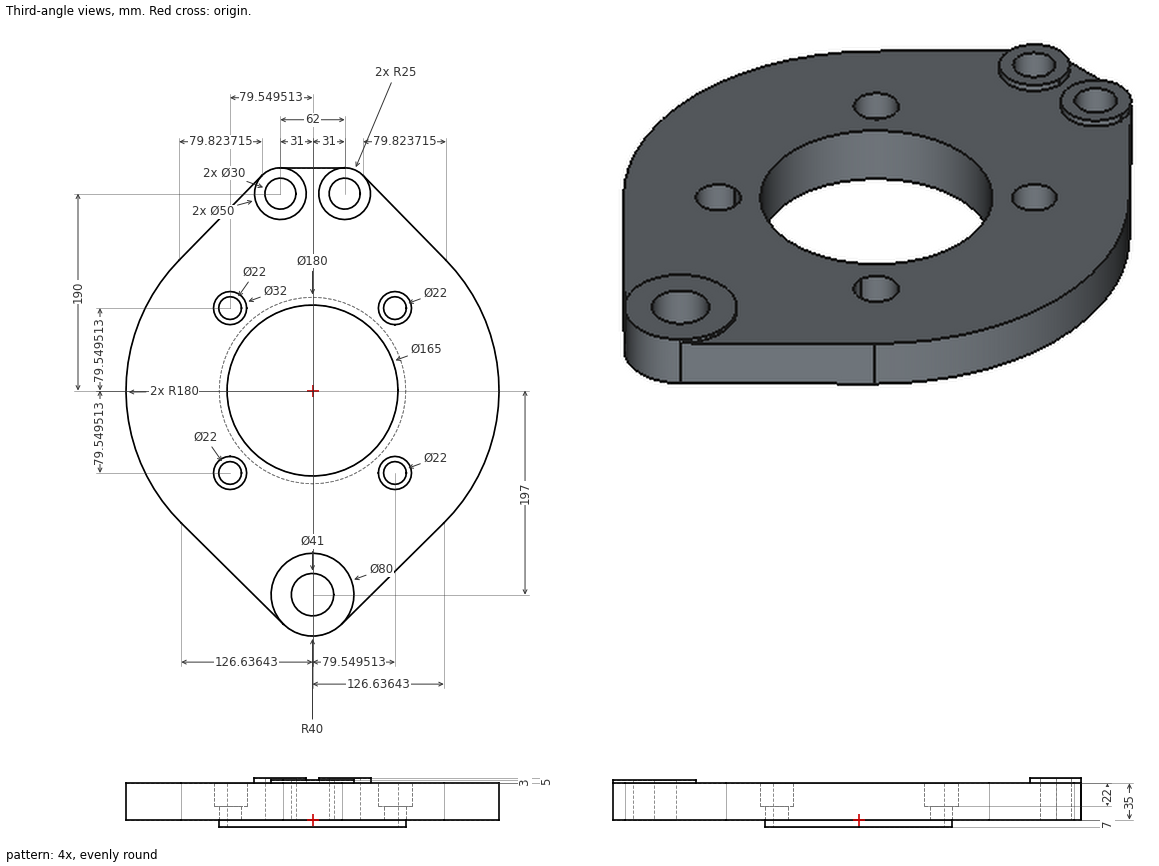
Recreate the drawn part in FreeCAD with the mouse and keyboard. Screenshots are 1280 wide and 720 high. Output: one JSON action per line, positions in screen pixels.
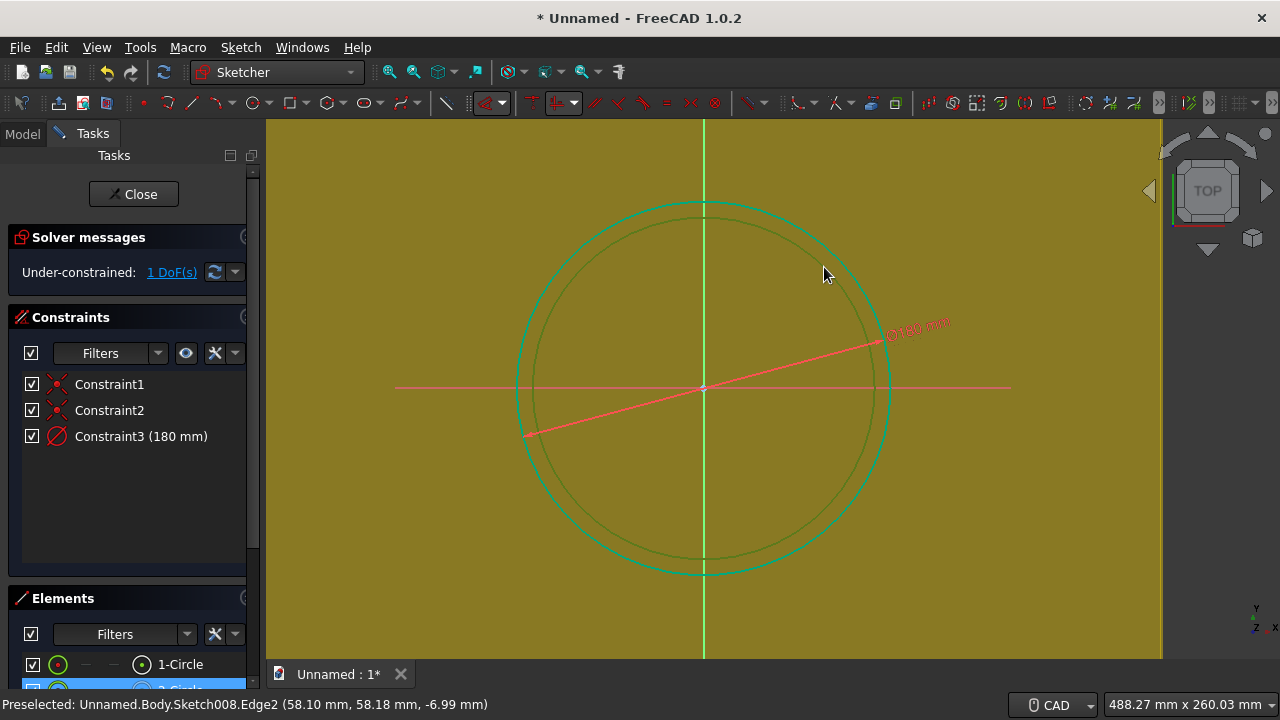
{"action": "key", "text": "k o"}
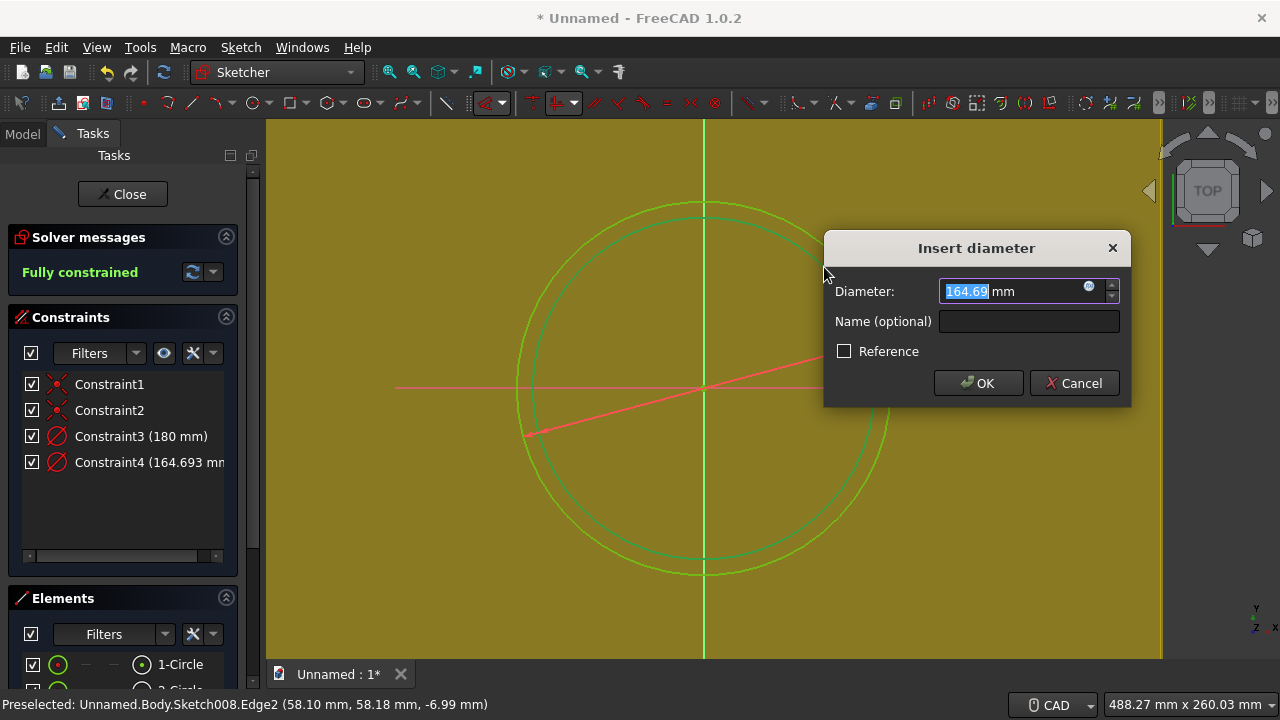
{"action": "type", "text": "165"}
{"action": "key", "text": "Return"}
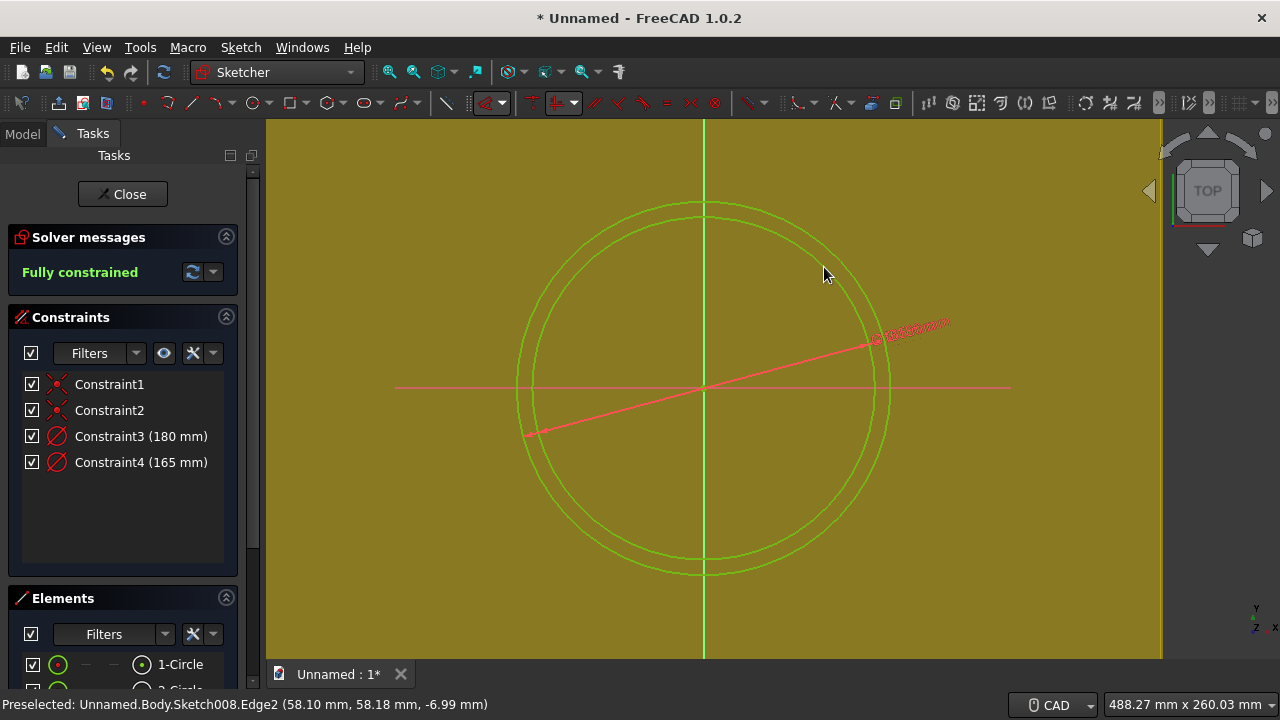
{"action": "left_click", "coordinate": [123, 194]}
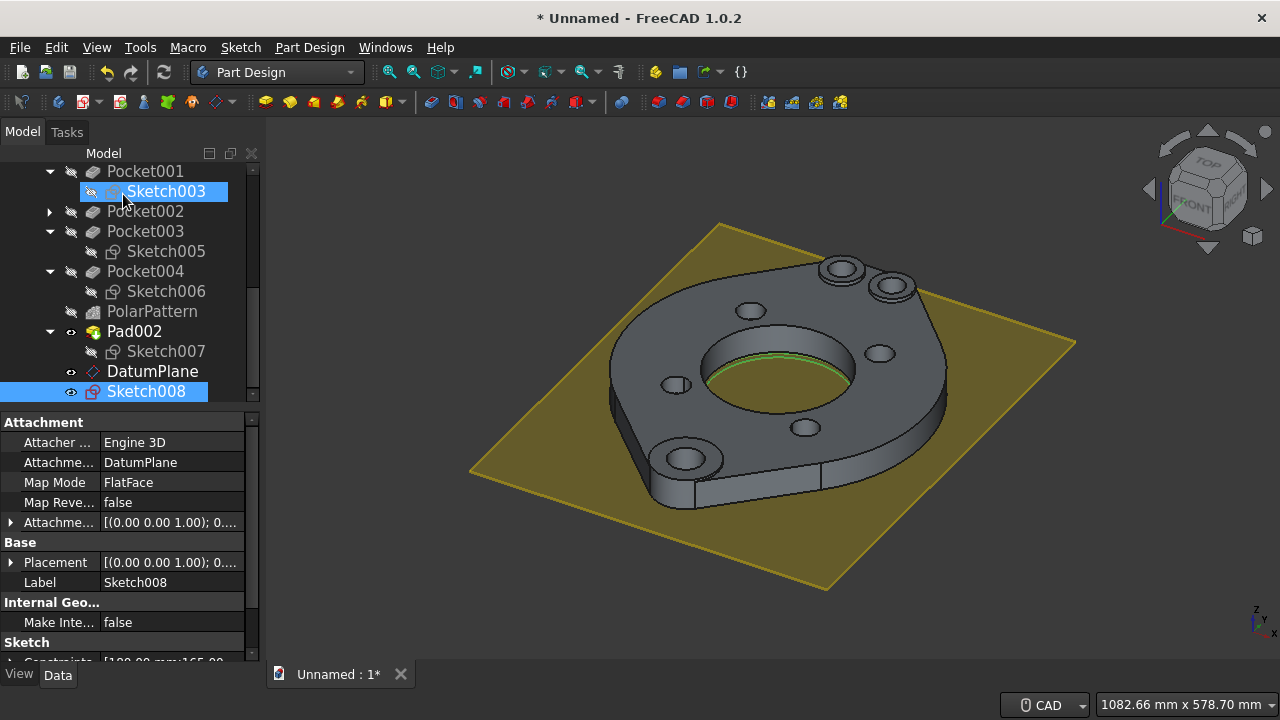
{"action": "left_click", "coordinate": [266, 102]}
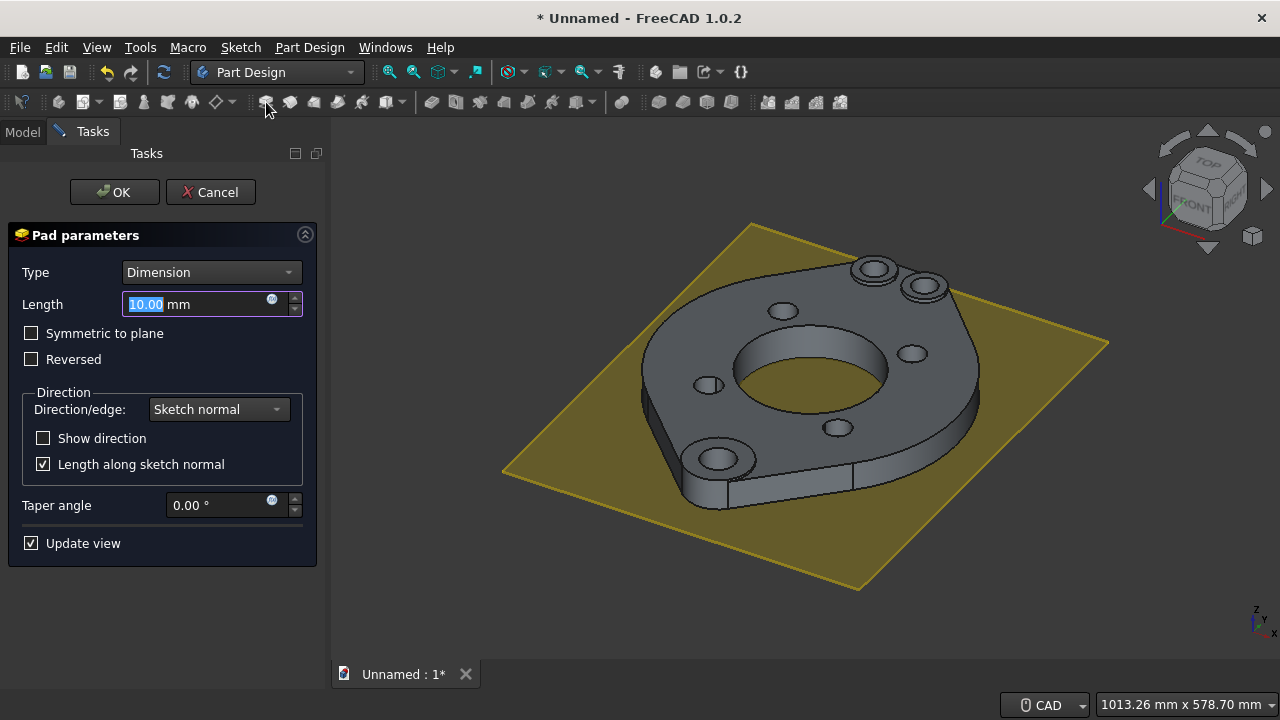
{"action": "type", "text": "7"}
{"action": "key", "text": "Tab"}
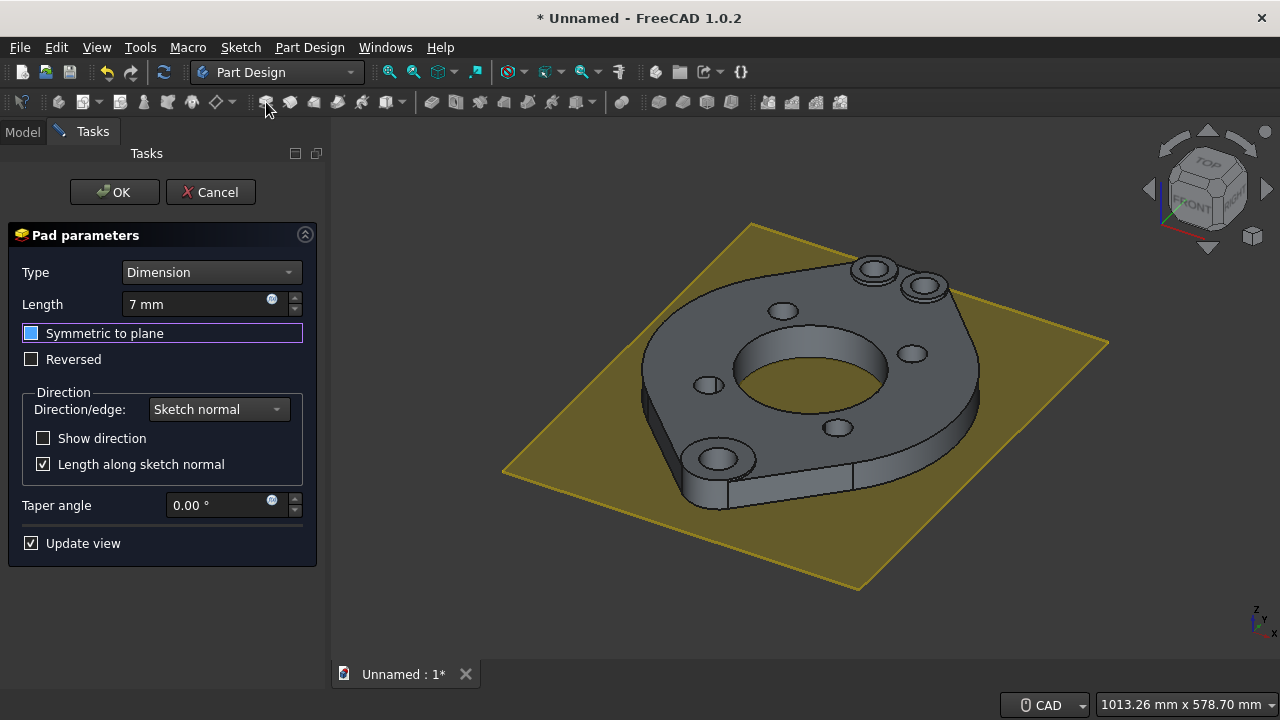
{"action": "left_click", "coordinate": [115, 192]}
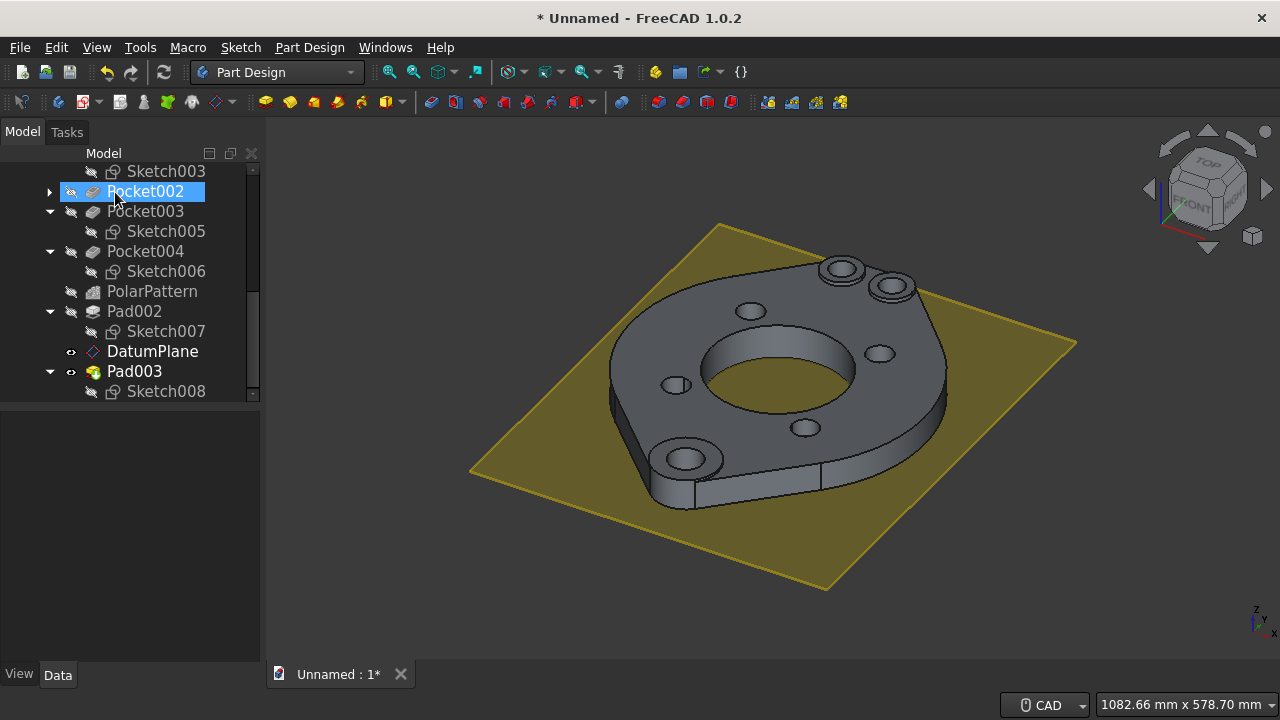
{"action": "left_click", "coordinate": [116, 352]}
{"action": "key", "text": "space"}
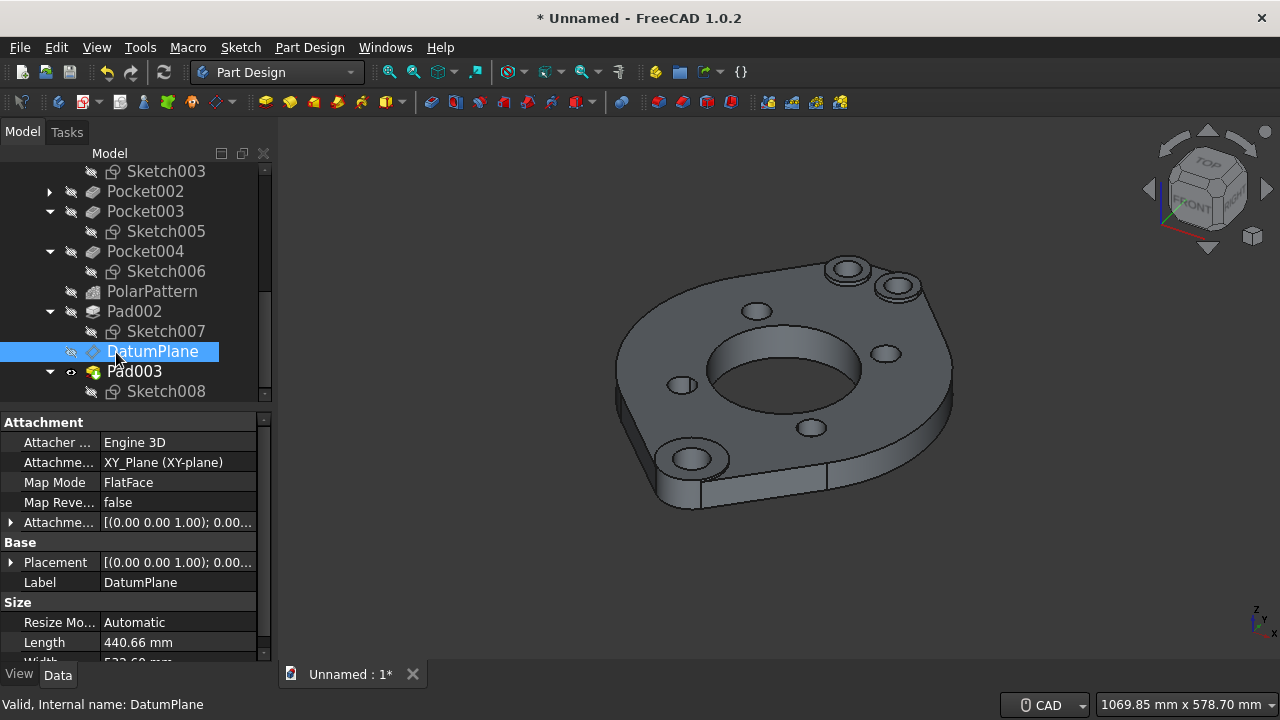
{"action": "key", "text": "0"}